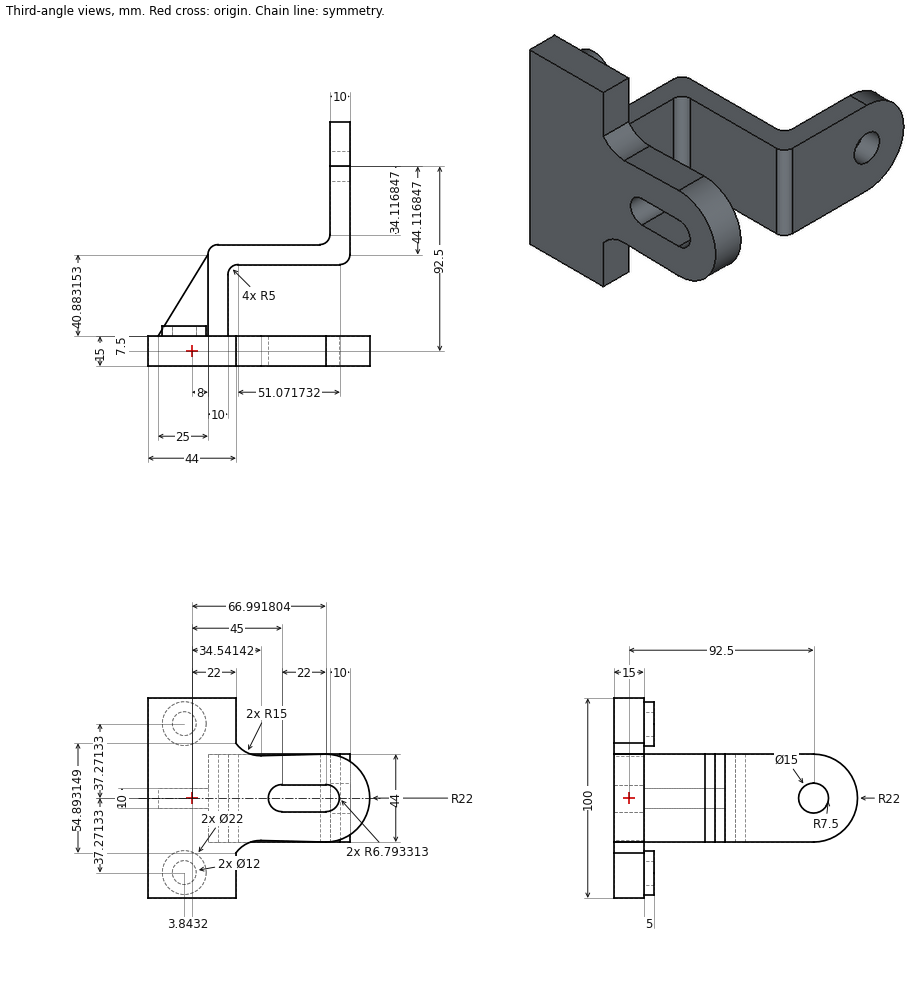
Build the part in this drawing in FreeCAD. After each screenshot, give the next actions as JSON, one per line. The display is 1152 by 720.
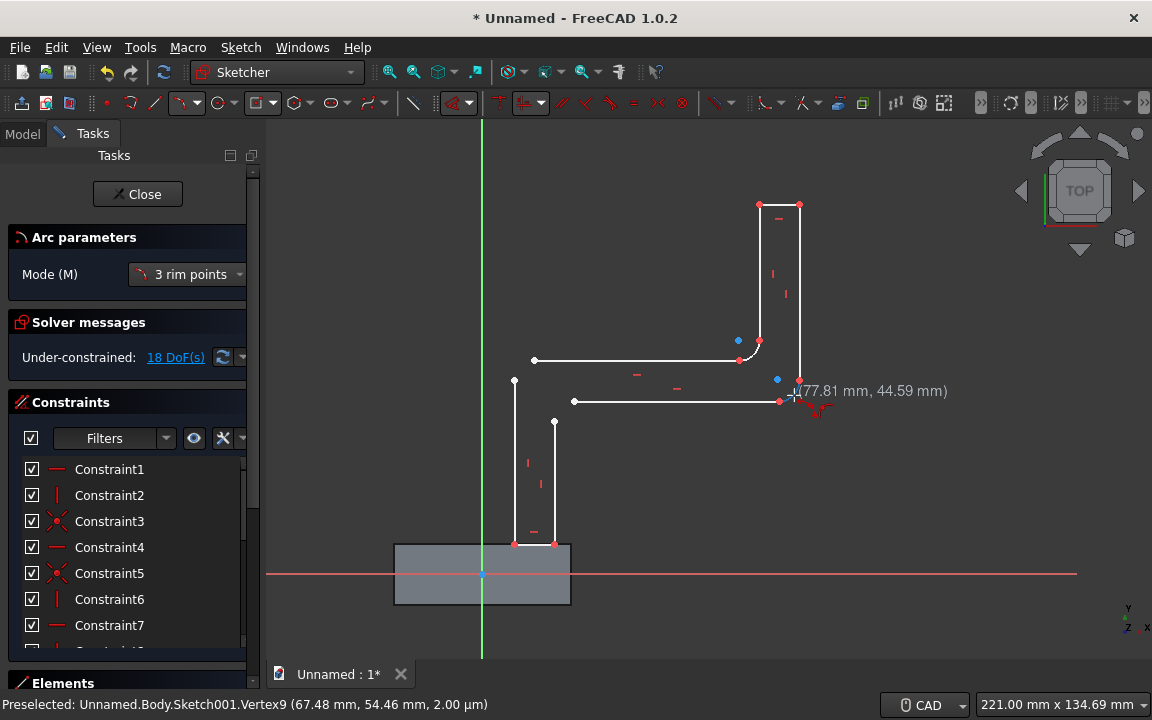
{"action": "left_click", "coordinate": [535, 361]}
{"action": "left_click", "coordinate": [515, 381]}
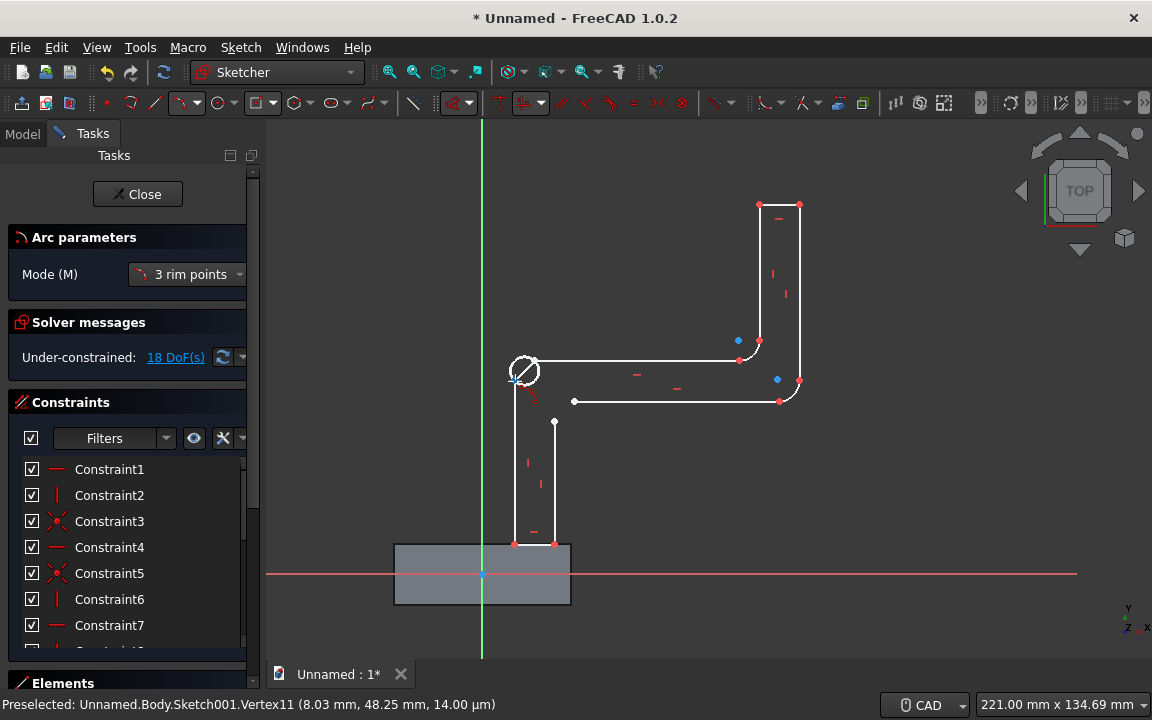
{"action": "scroll", "coordinate": [520, 366], "scroll_direction": "up", "scroll_amount": 5}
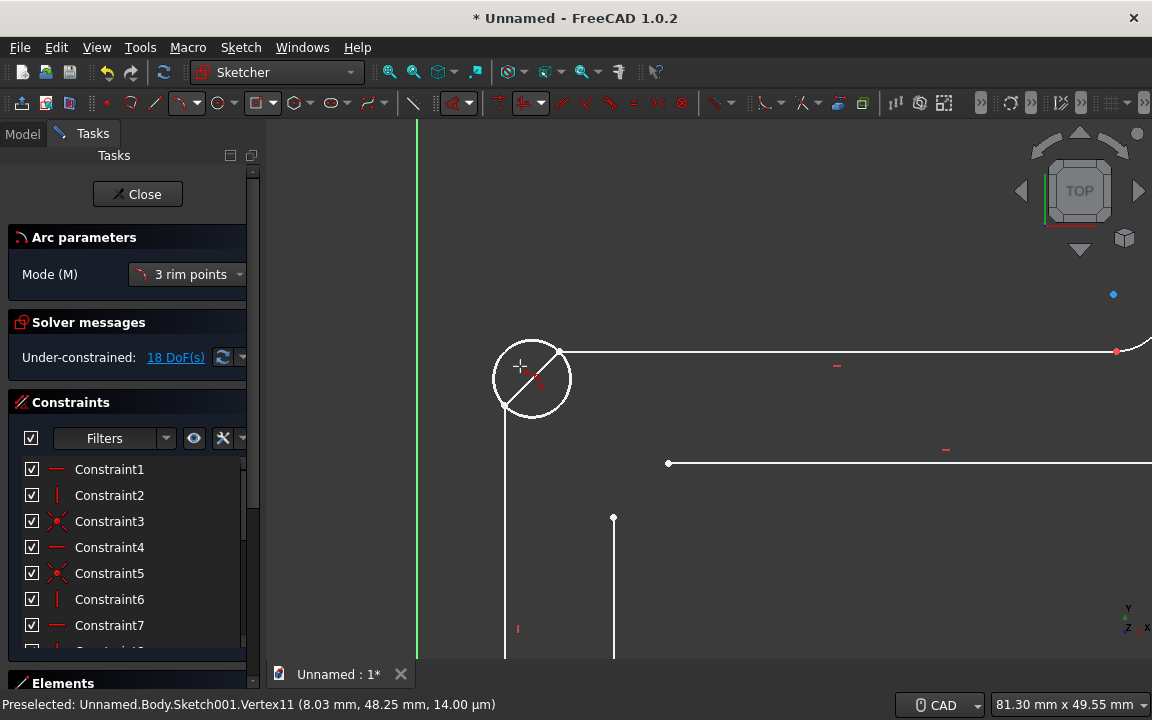
{"action": "left_click", "coordinate": [521, 366]}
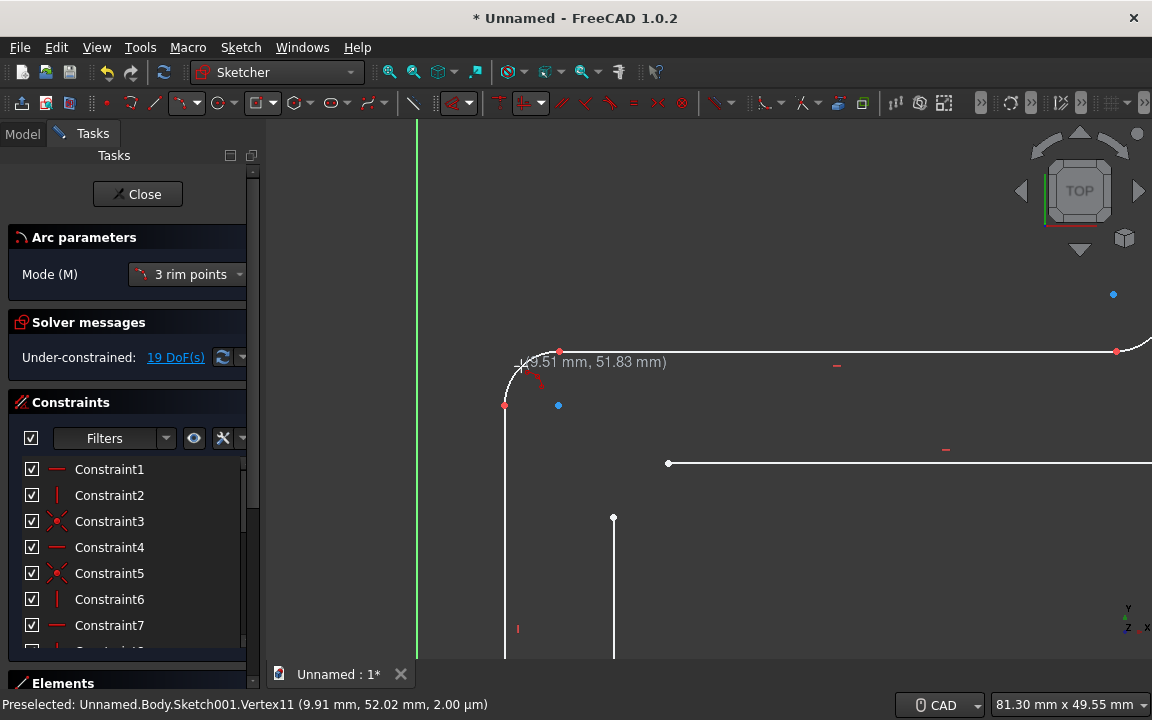
{"action": "left_click", "coordinate": [614, 517]}
{"action": "left_click", "coordinate": [668, 463]}
{"action": "left_click", "coordinate": [629, 475]}
{"action": "key", "text": "Escape"}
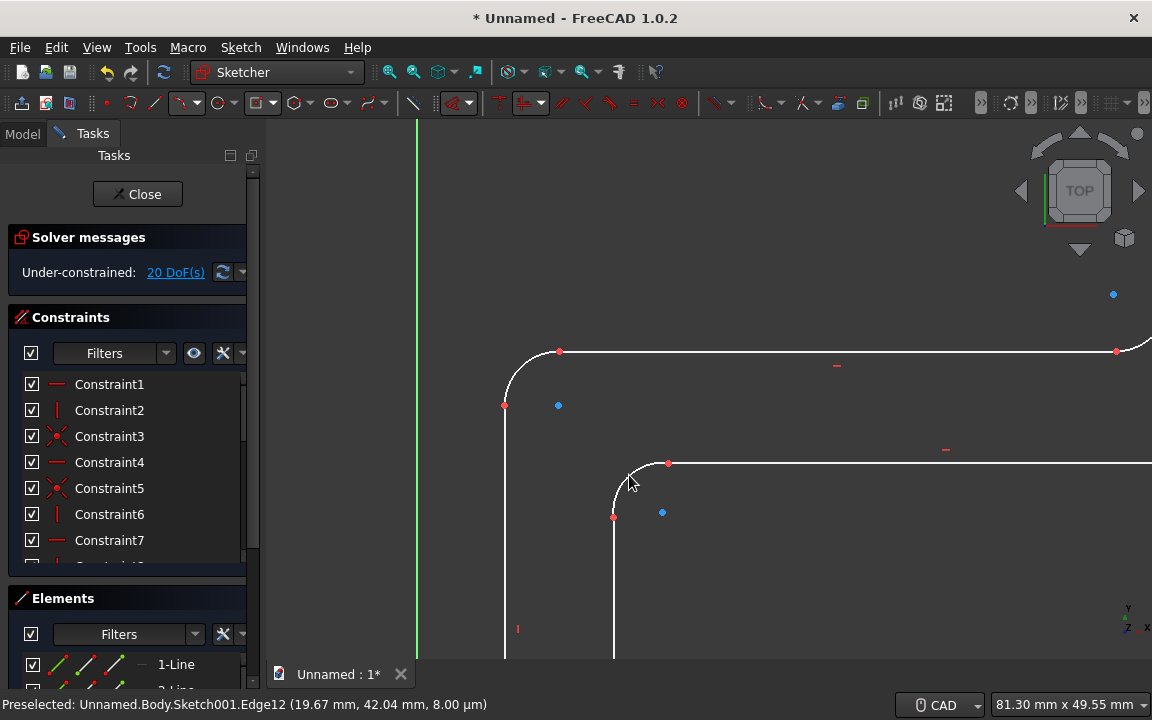
{"action": "left_click", "coordinate": [835, 463]}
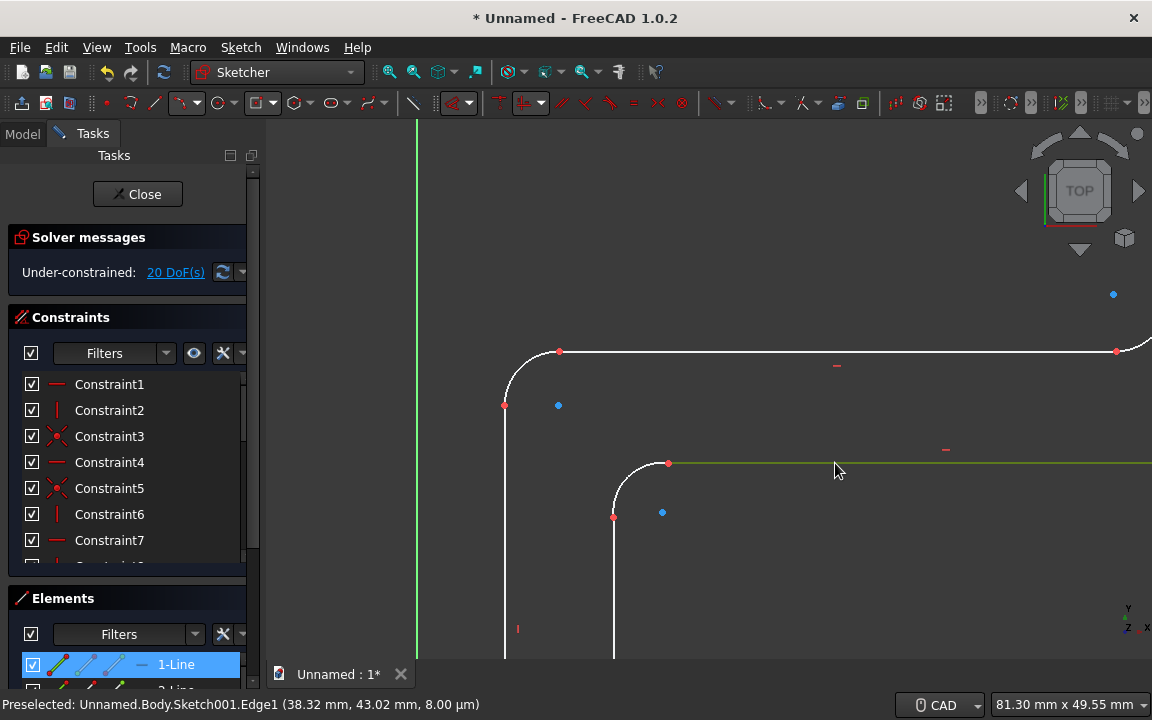
{"action": "scroll", "coordinate": [520, 366], "scroll_direction": "down", "scroll_amount": 5}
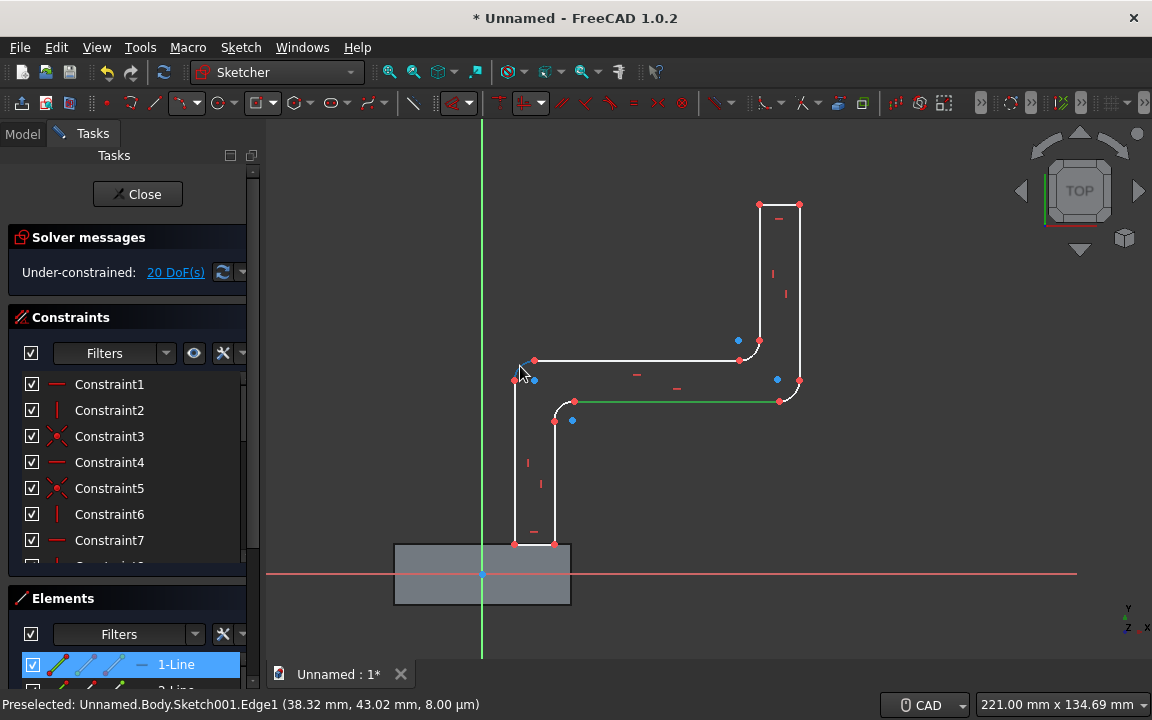
{"action": "scroll", "coordinate": [789, 399], "scroll_direction": "up", "scroll_amount": 2}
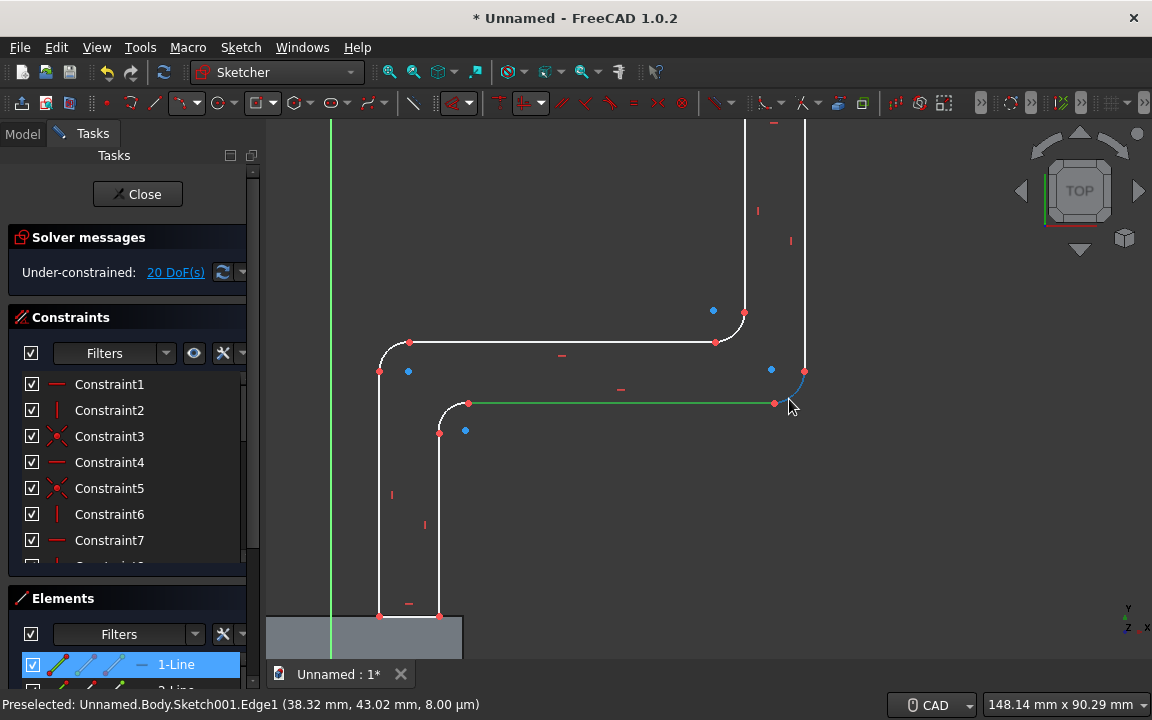
{"action": "left_click", "coordinate": [788, 399]}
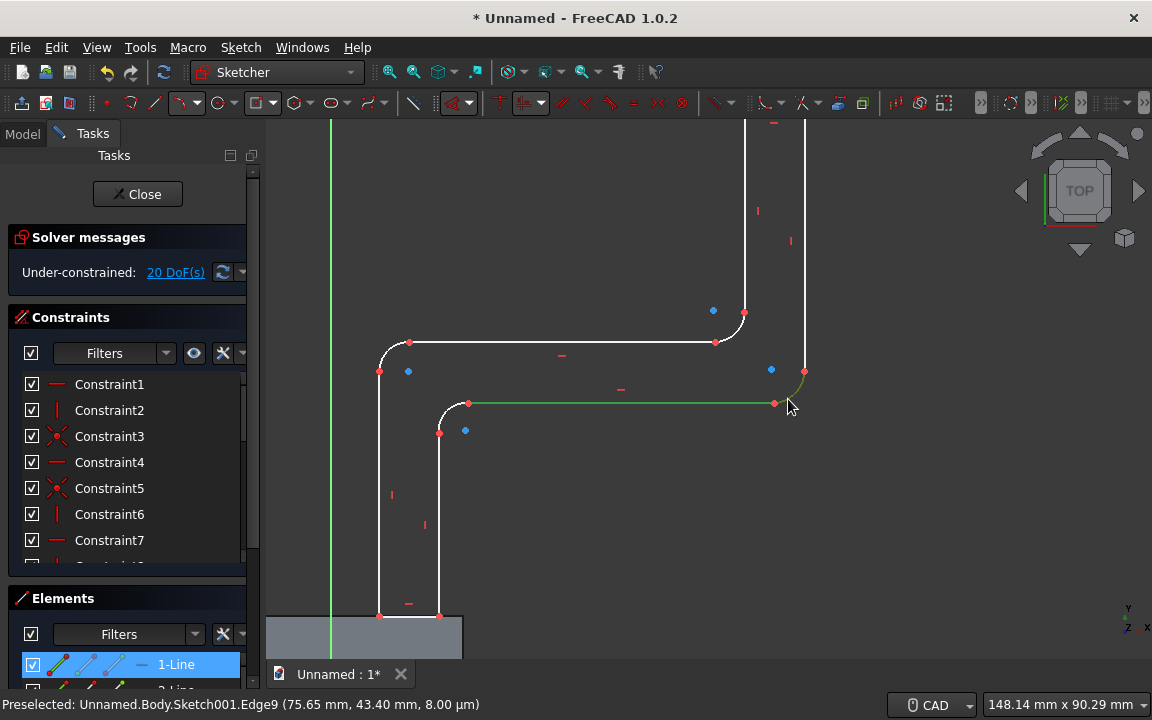
{"action": "left_click", "coordinate": [610, 104]}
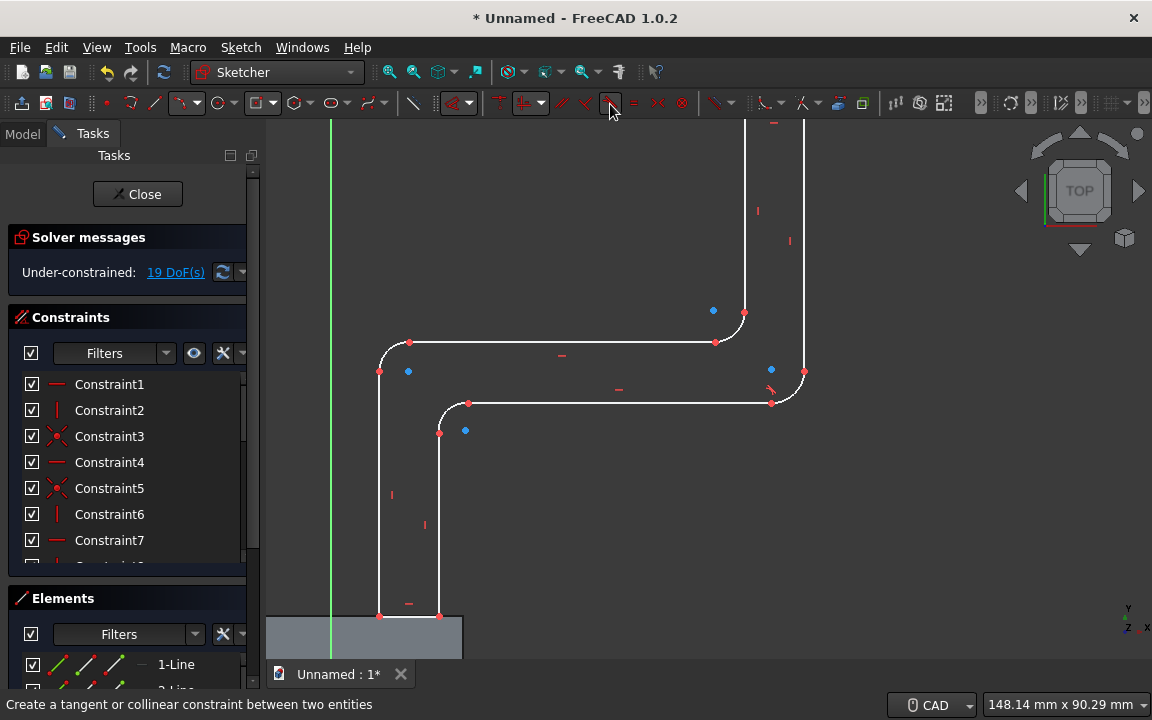
{"action": "left_click", "coordinate": [560, 403]}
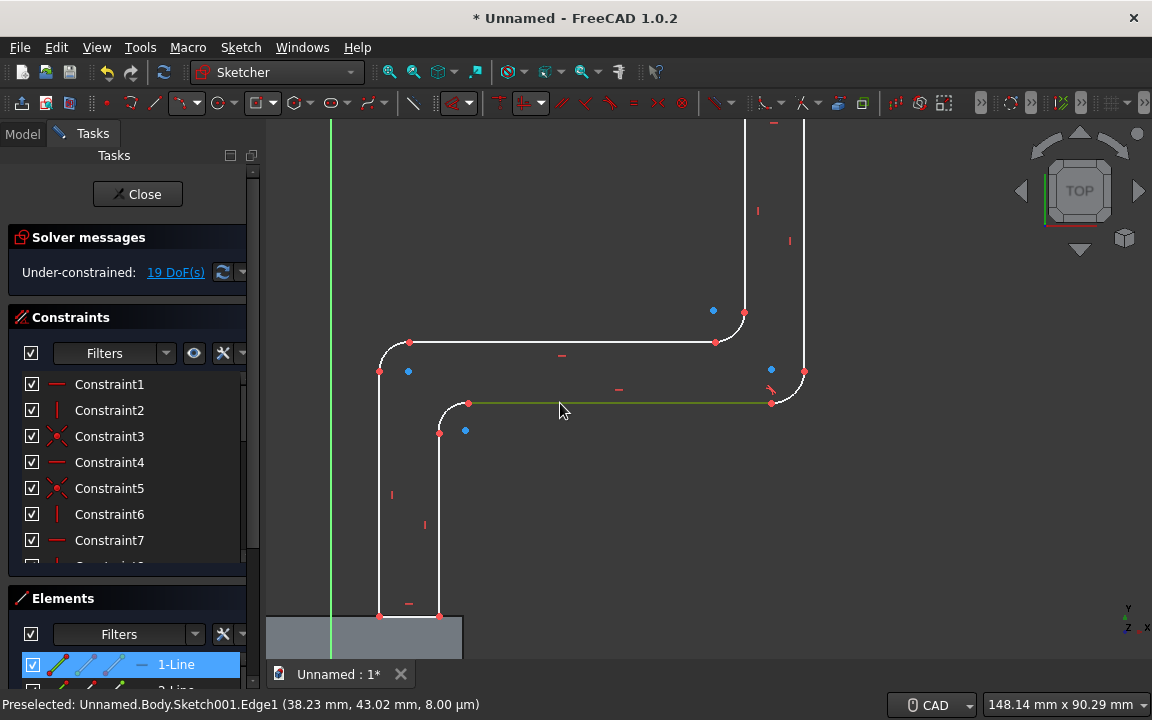
{"action": "left_click", "coordinate": [455, 405]}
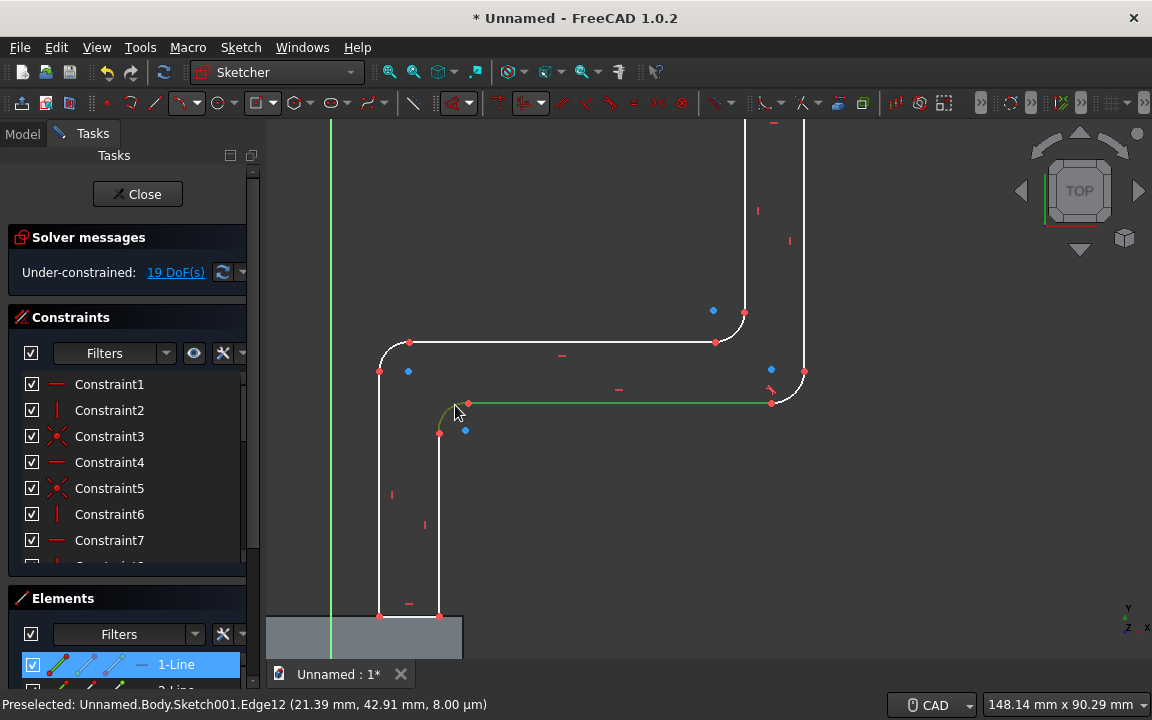
{"action": "left_click", "coordinate": [610, 104]}